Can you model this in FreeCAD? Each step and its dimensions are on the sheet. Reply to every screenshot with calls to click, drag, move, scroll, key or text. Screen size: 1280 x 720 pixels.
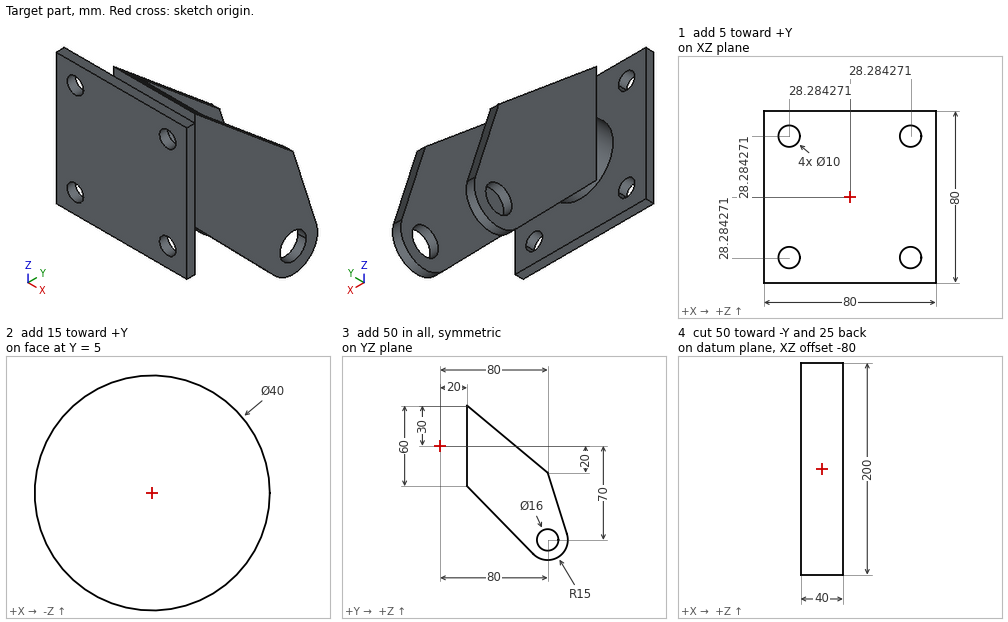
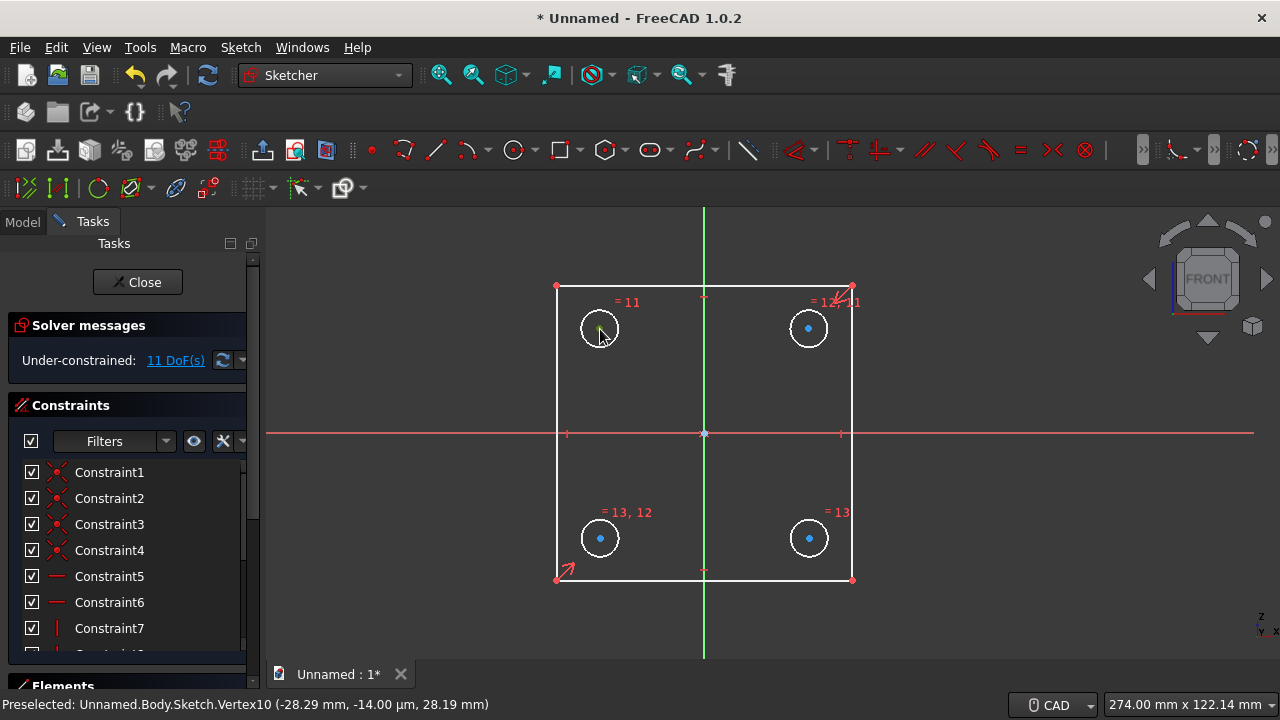
click(809, 329)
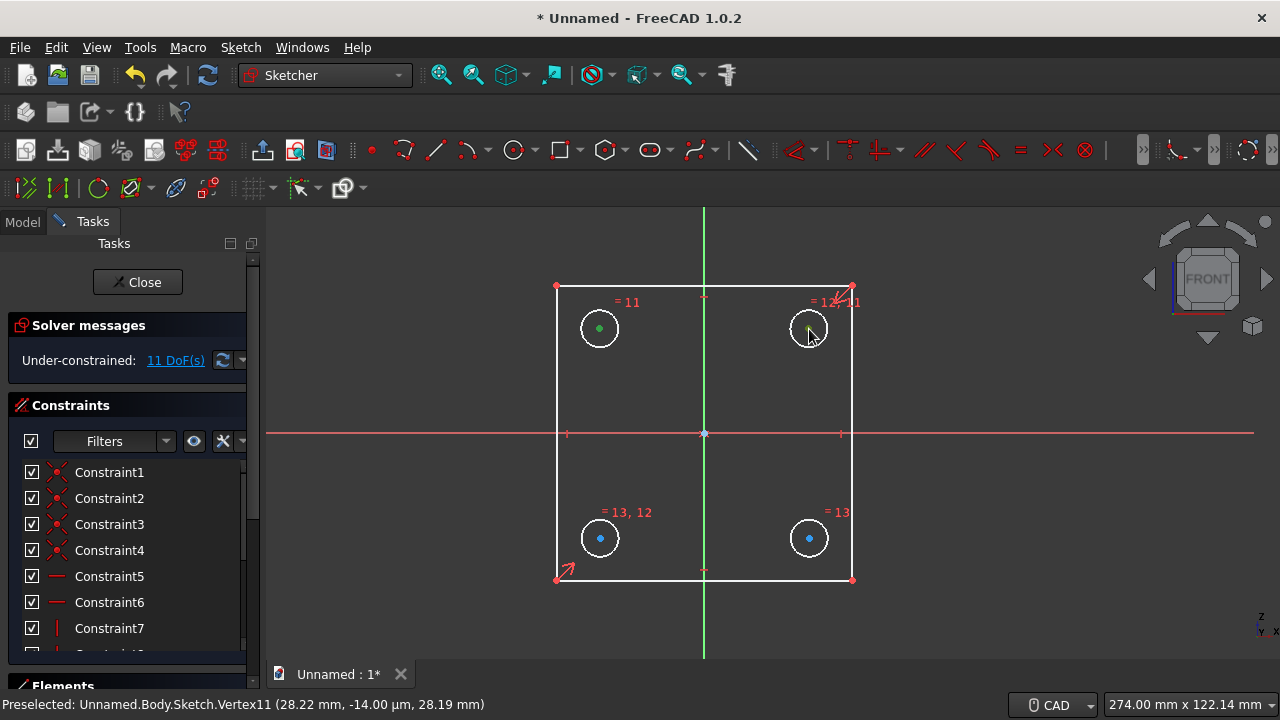
click(902, 150)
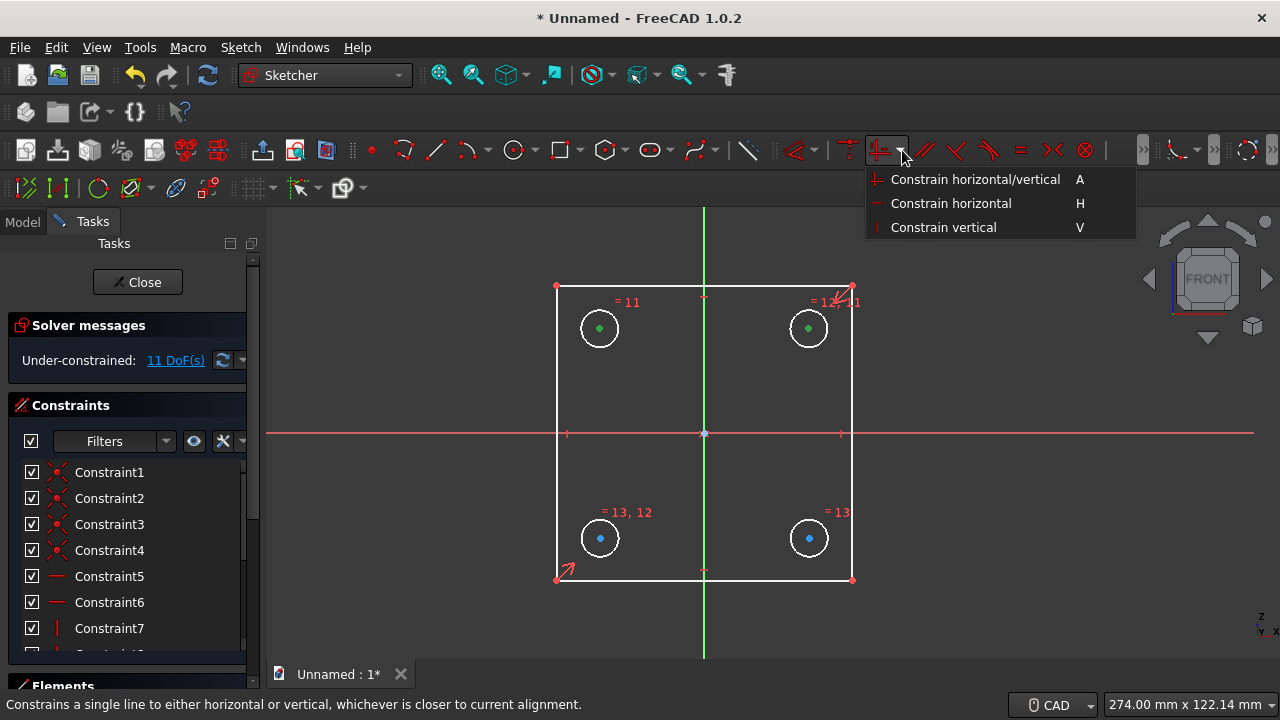
click(1001, 203)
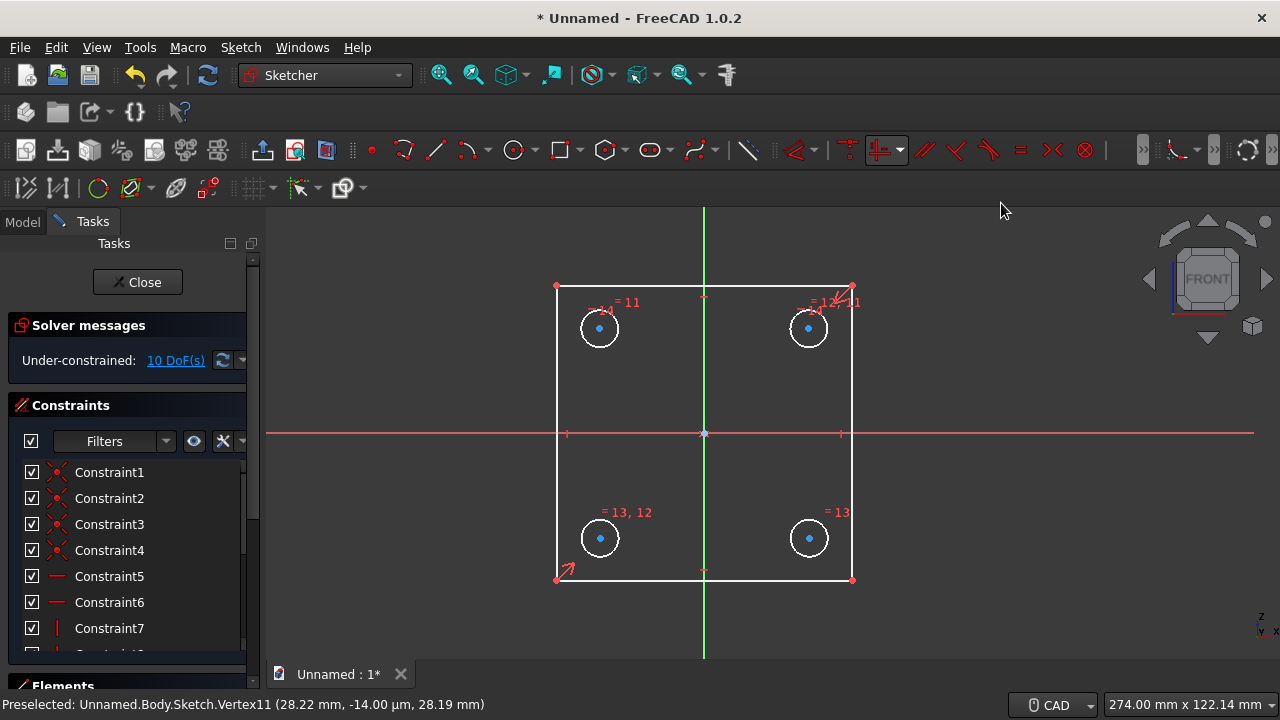
click(600, 329)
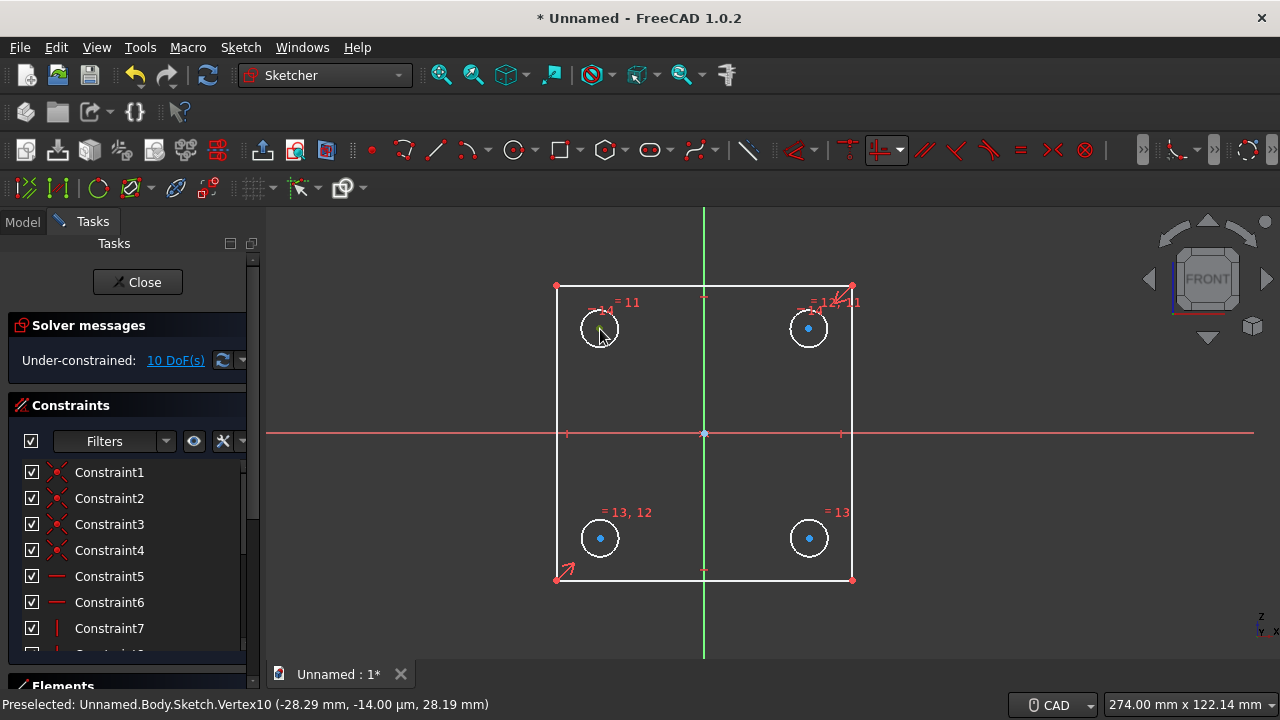
click(600, 538)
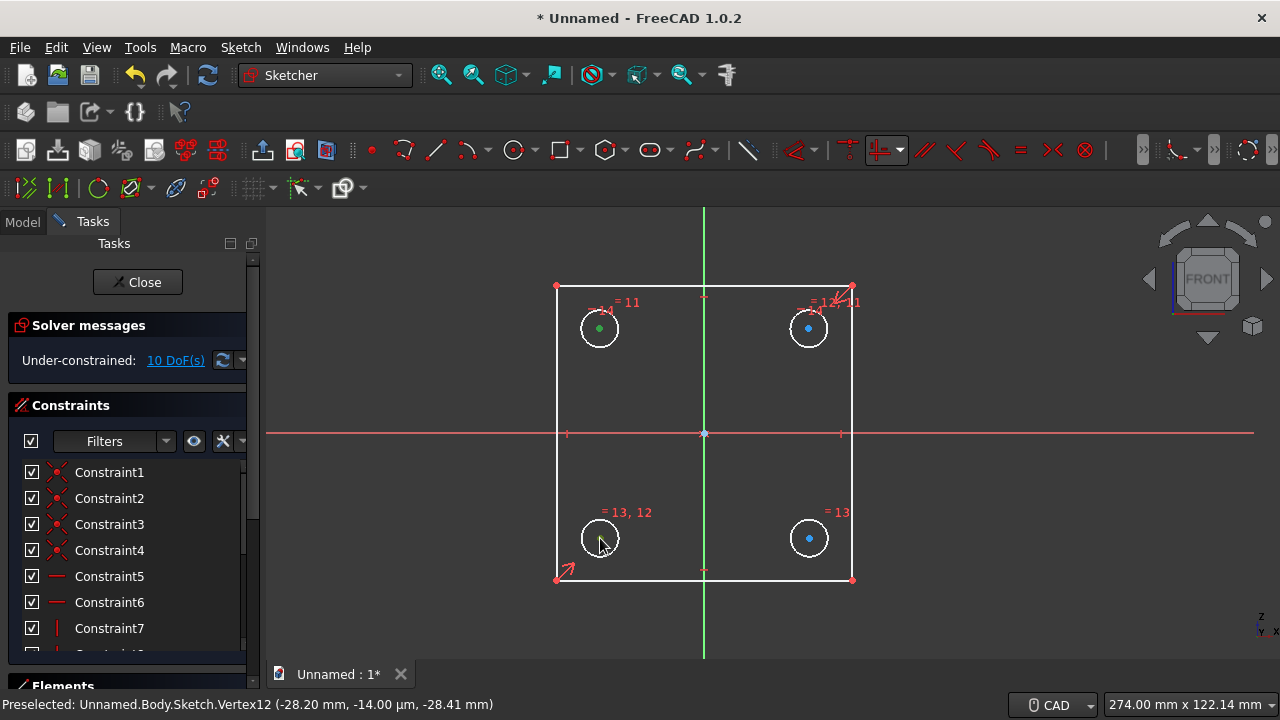
click(902, 150)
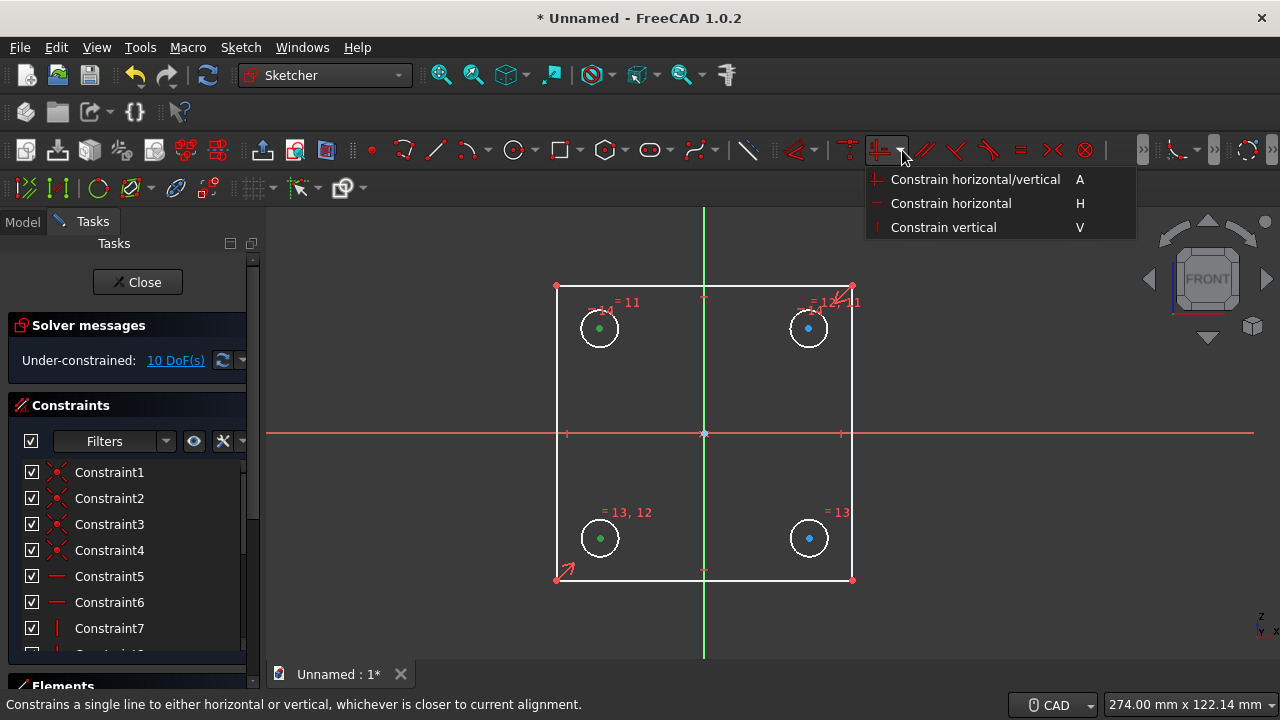
click(1001, 227)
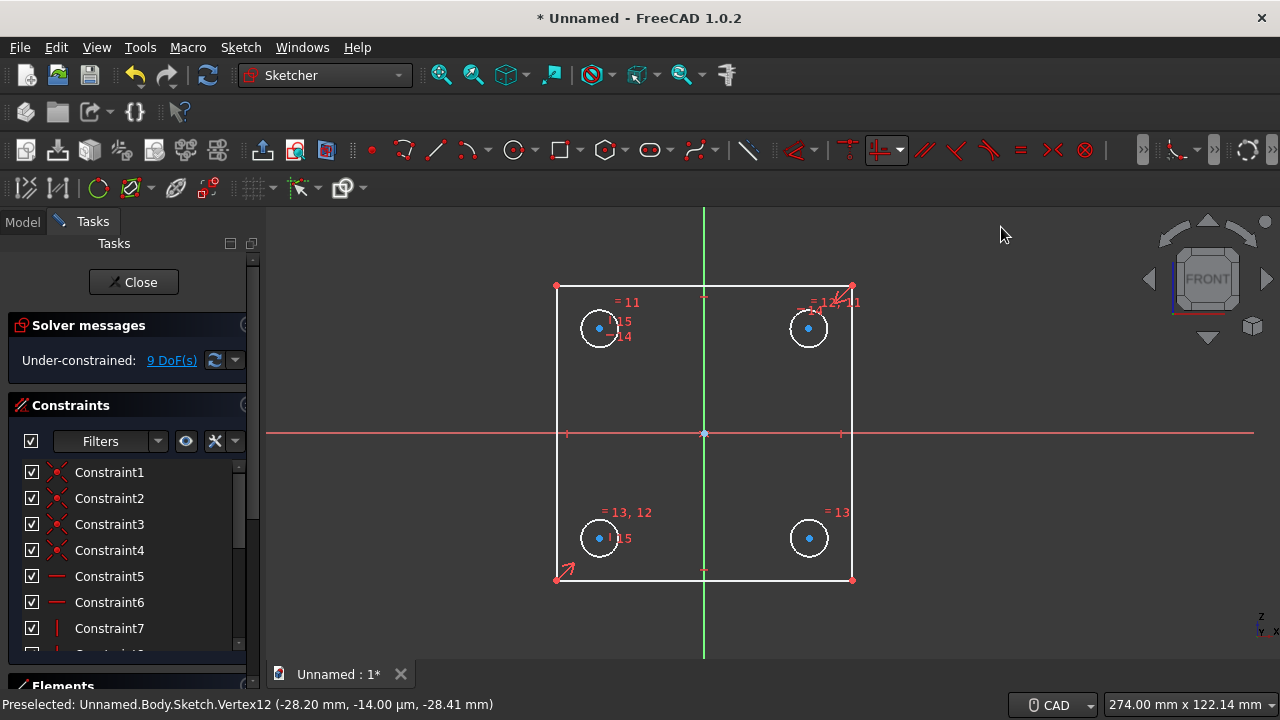
click(809, 329)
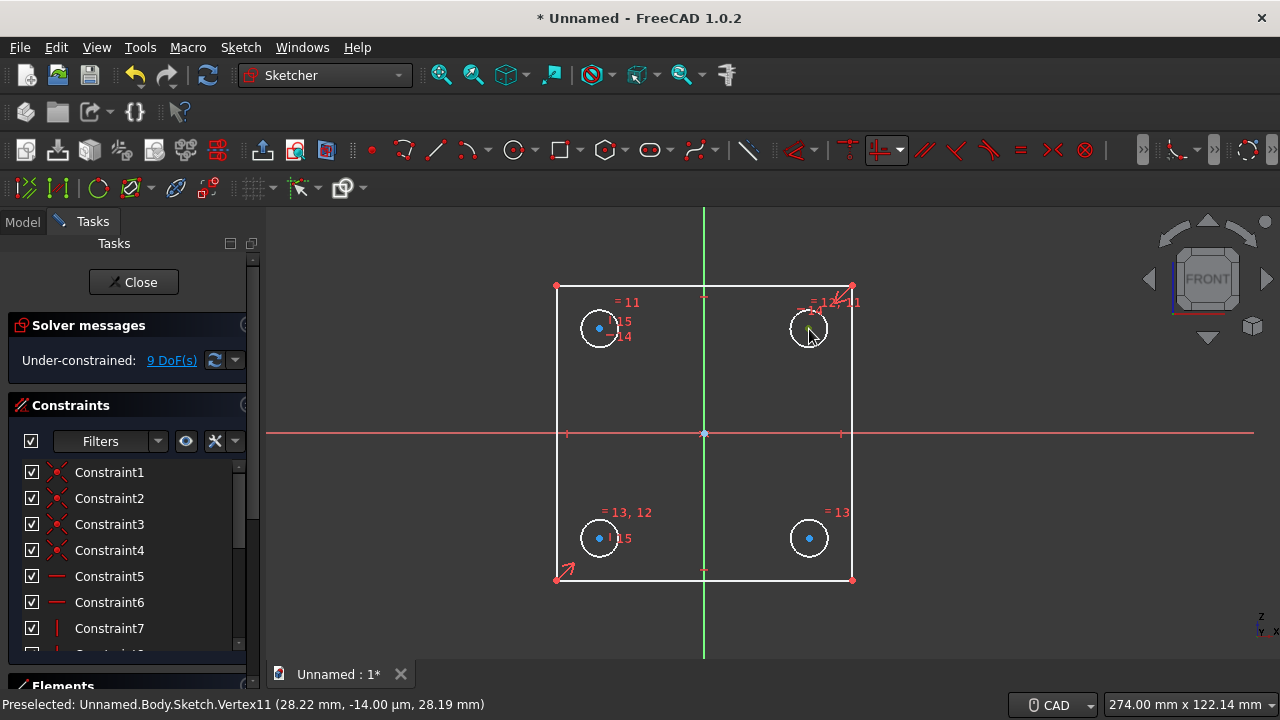
click(809, 538)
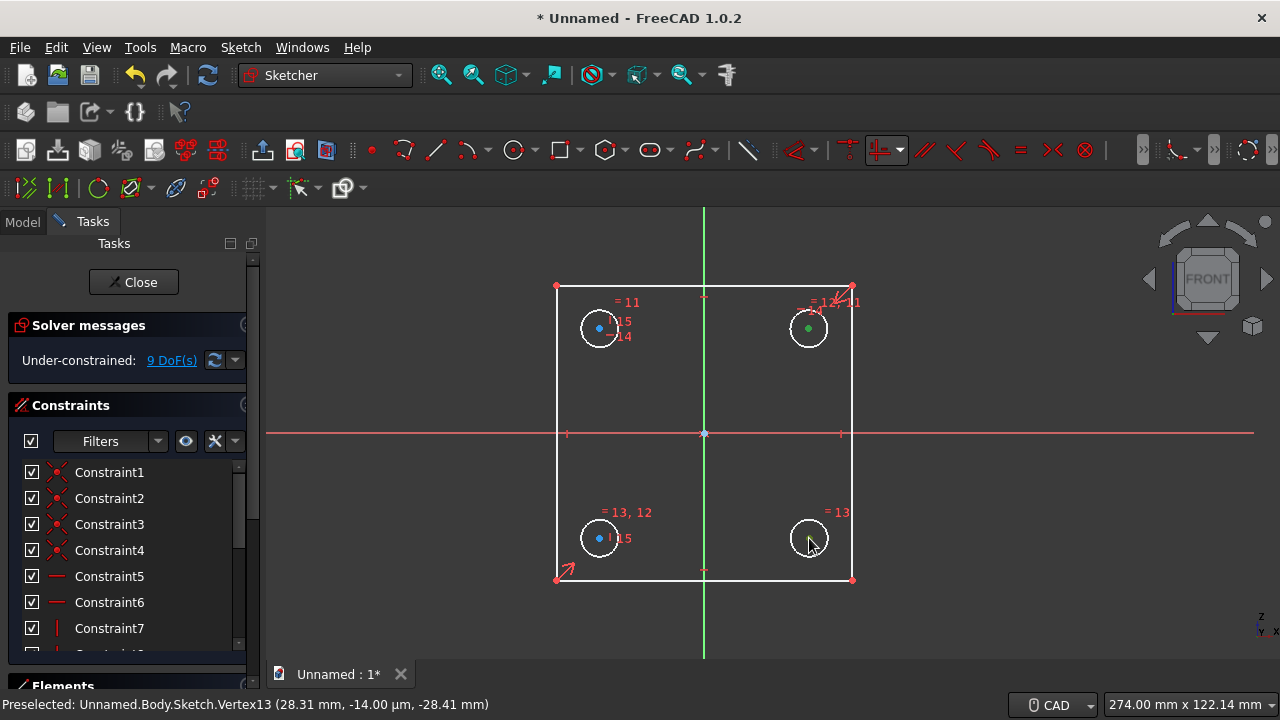
key(v)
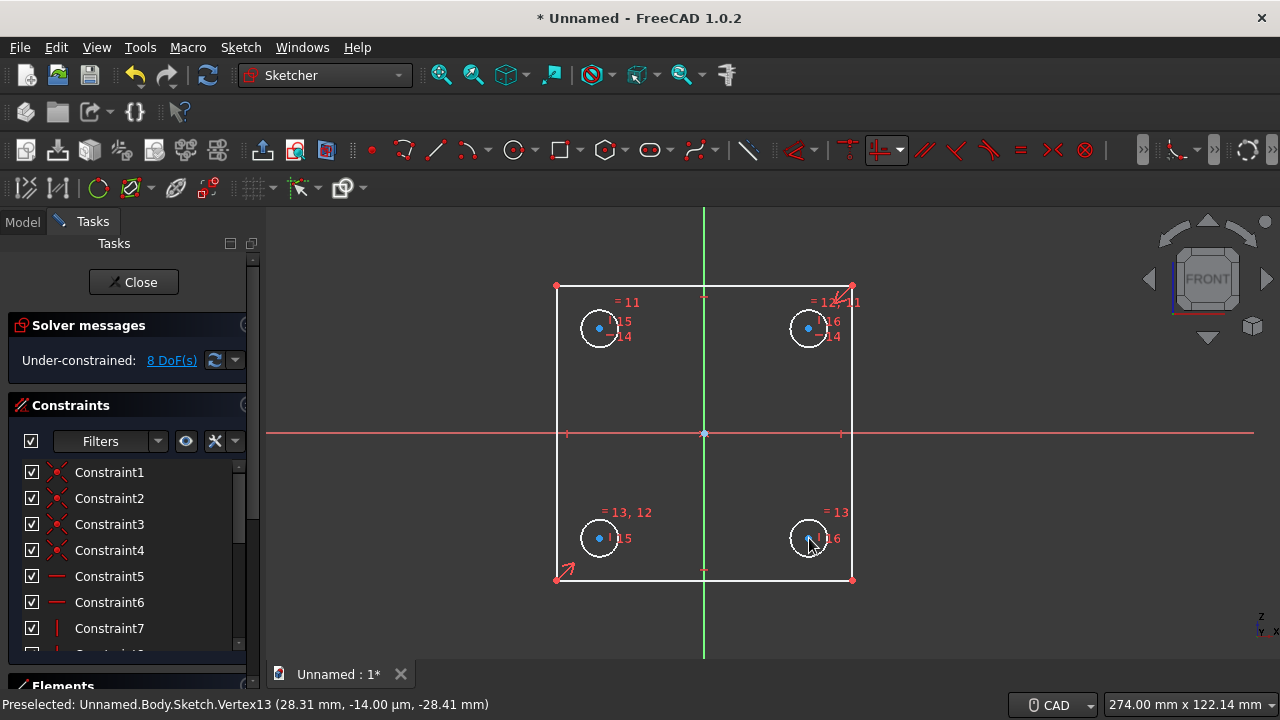
click(600, 538)